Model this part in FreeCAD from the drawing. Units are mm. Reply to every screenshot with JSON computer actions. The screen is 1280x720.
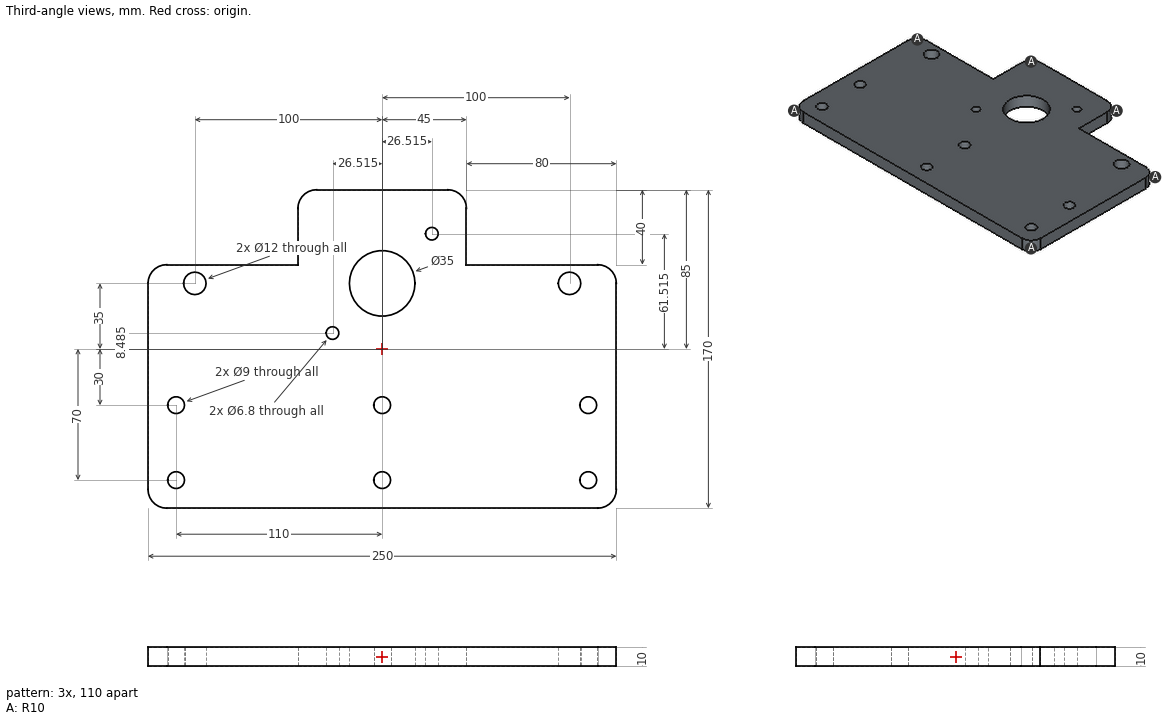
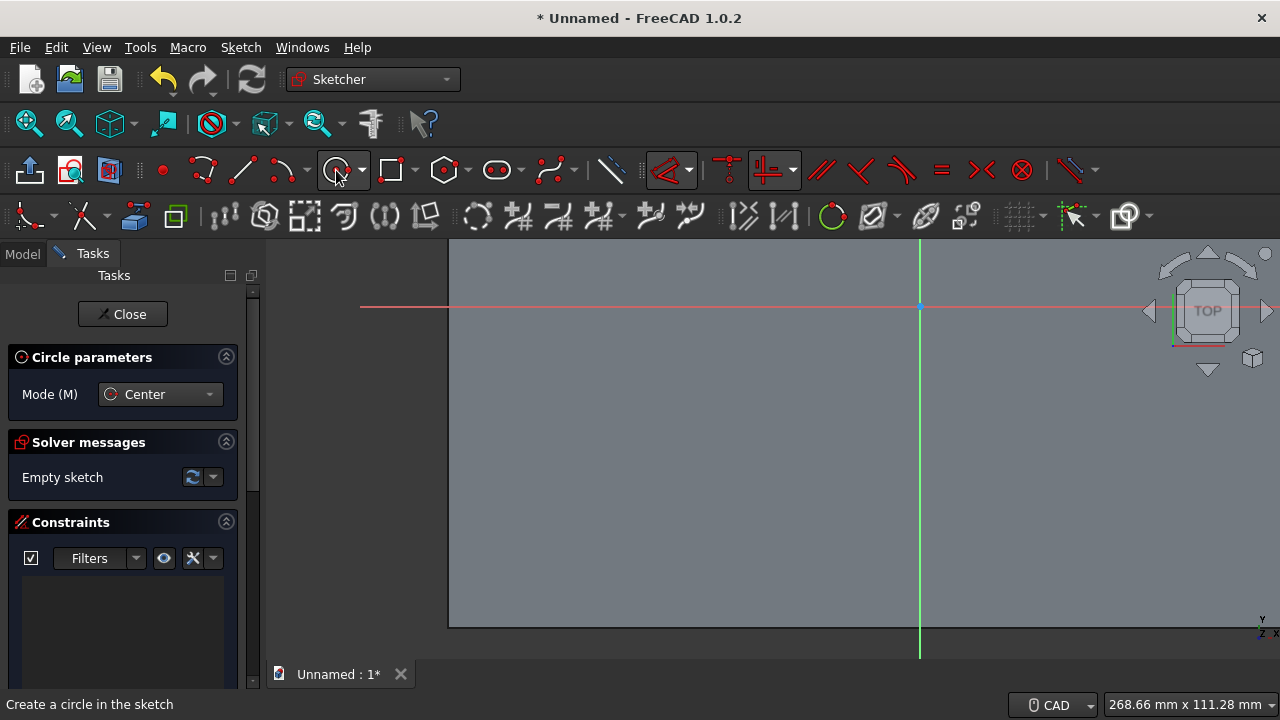
{"action": "scroll", "coordinate": [505, 420], "scroll_direction": "up", "scroll_amount": 2}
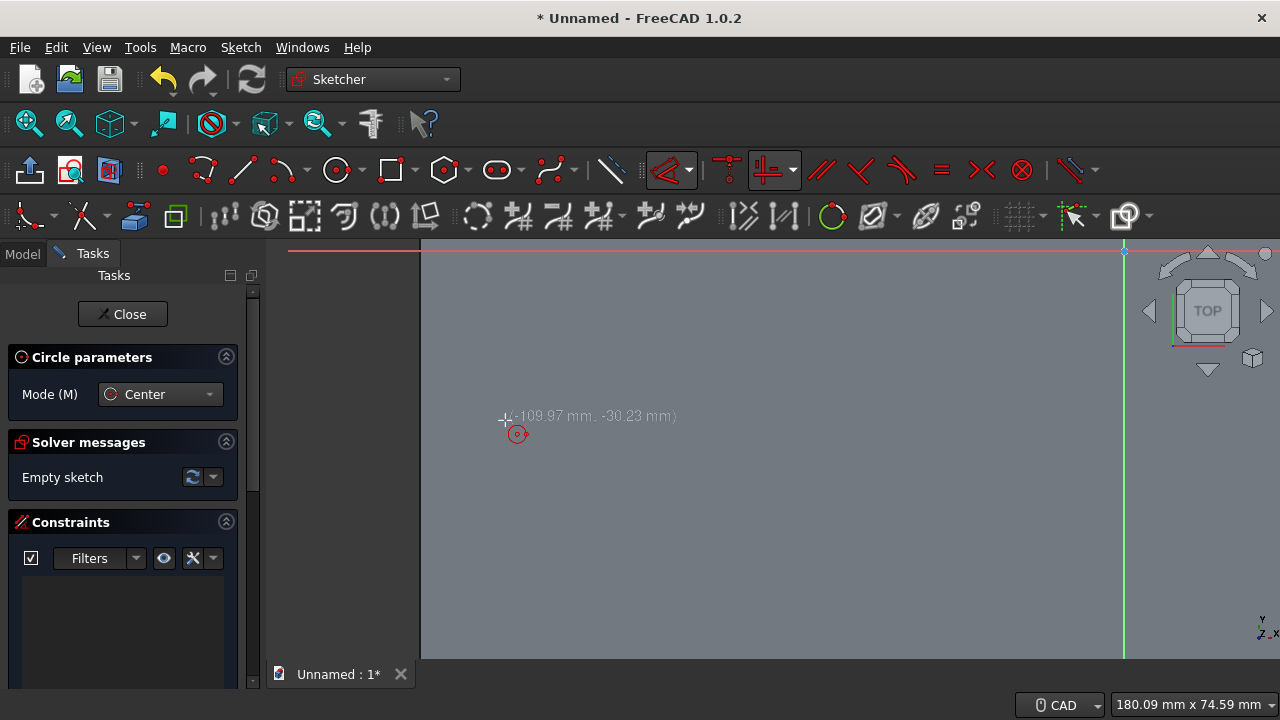
{"action": "left_click", "coordinate": [505, 420]}
{"action": "mouse_move", "coordinate": [523, 402]}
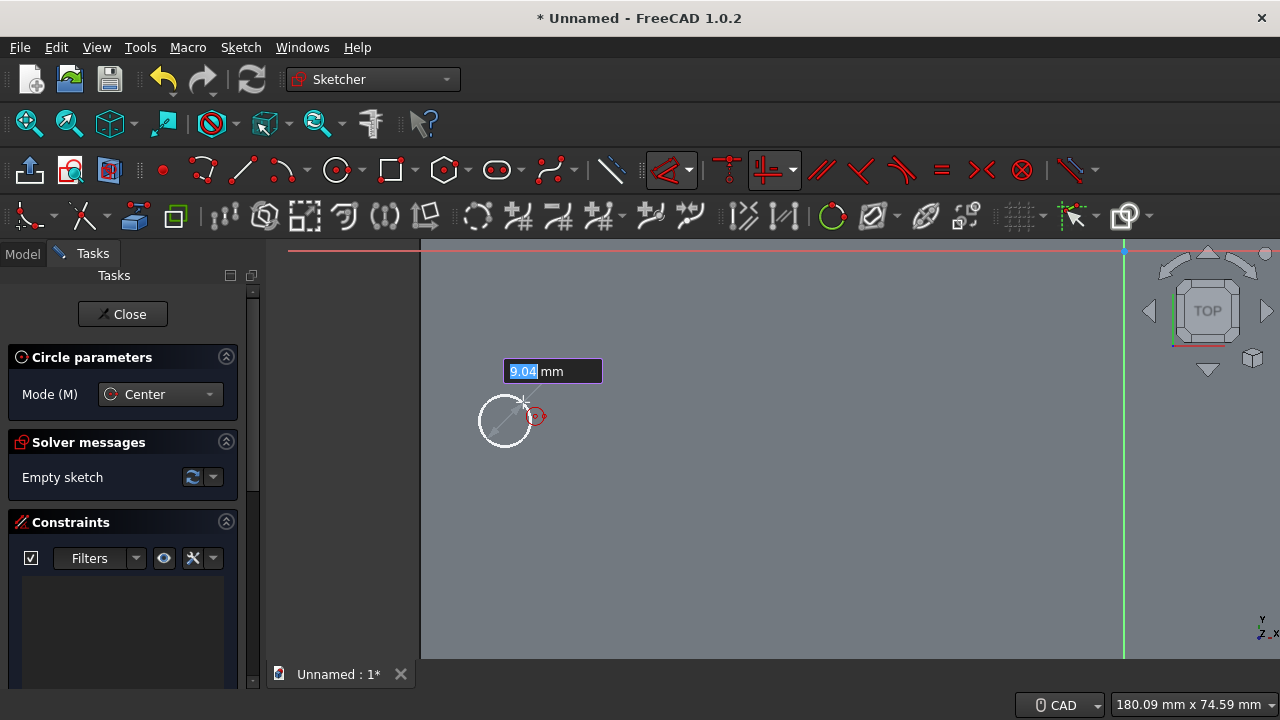
{"action": "type", "text": "9"}
{"action": "key", "text": "Return"}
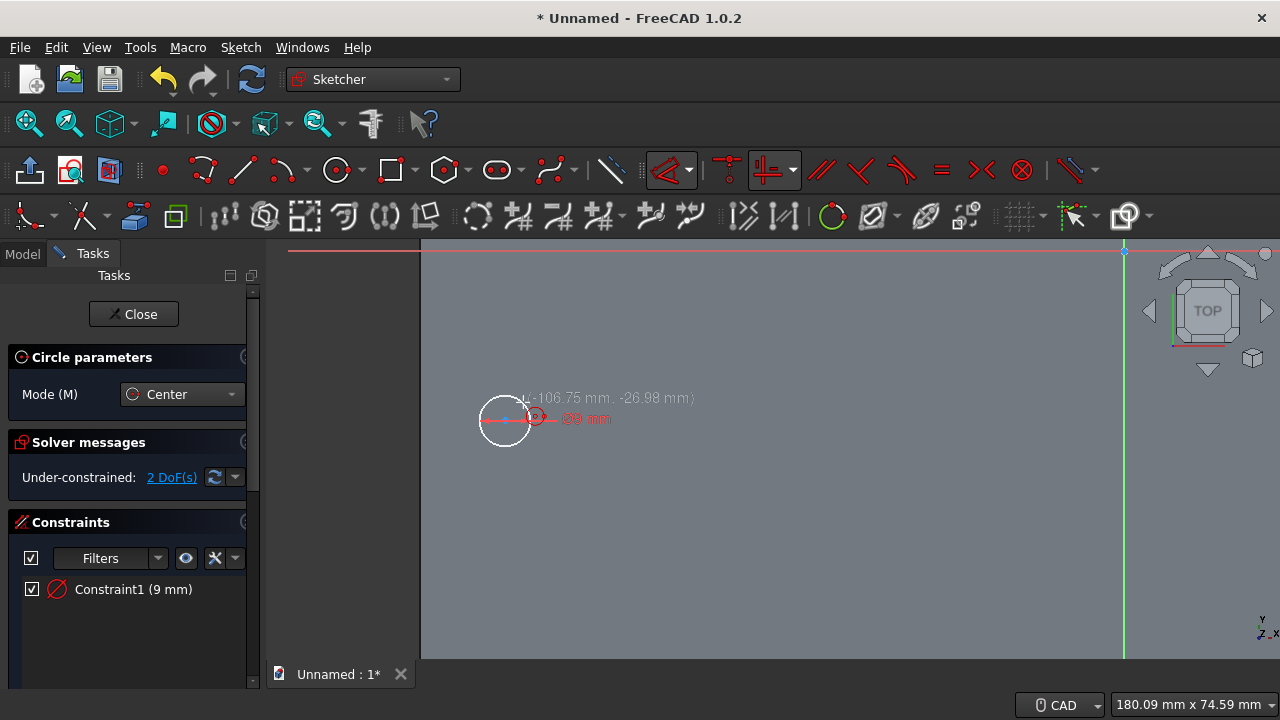
{"action": "scroll", "coordinate": [507, 425], "scroll_direction": "down", "scroll_amount": 2}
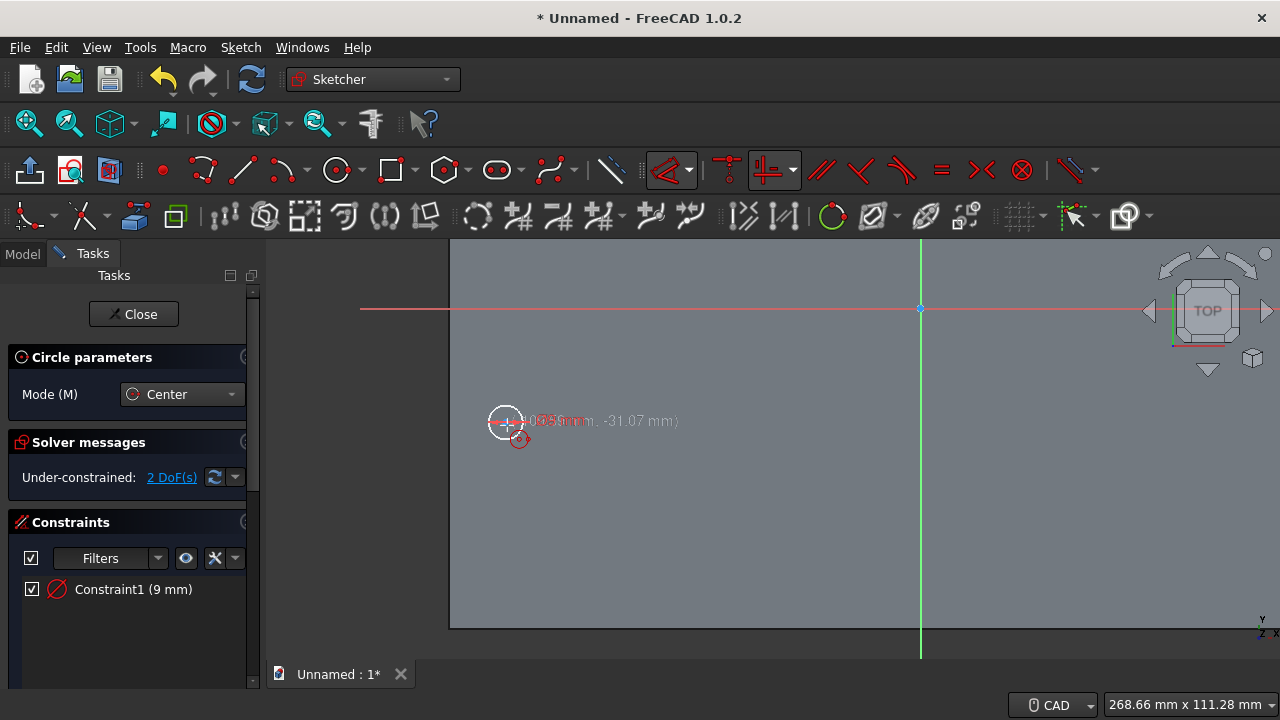
{"action": "scroll", "coordinate": [506, 573], "scroll_direction": "up", "scroll_amount": 2}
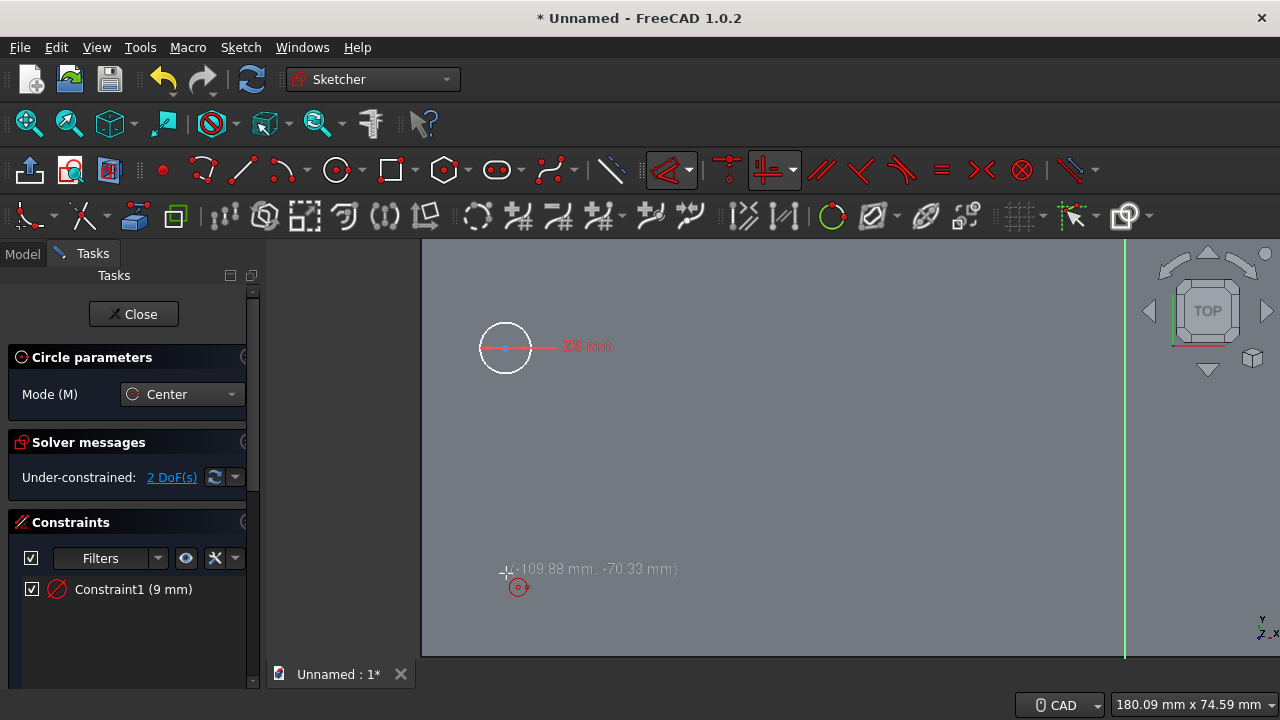
{"action": "left_click", "coordinate": [505, 572]}
{"action": "mouse_move", "coordinate": [523, 554]}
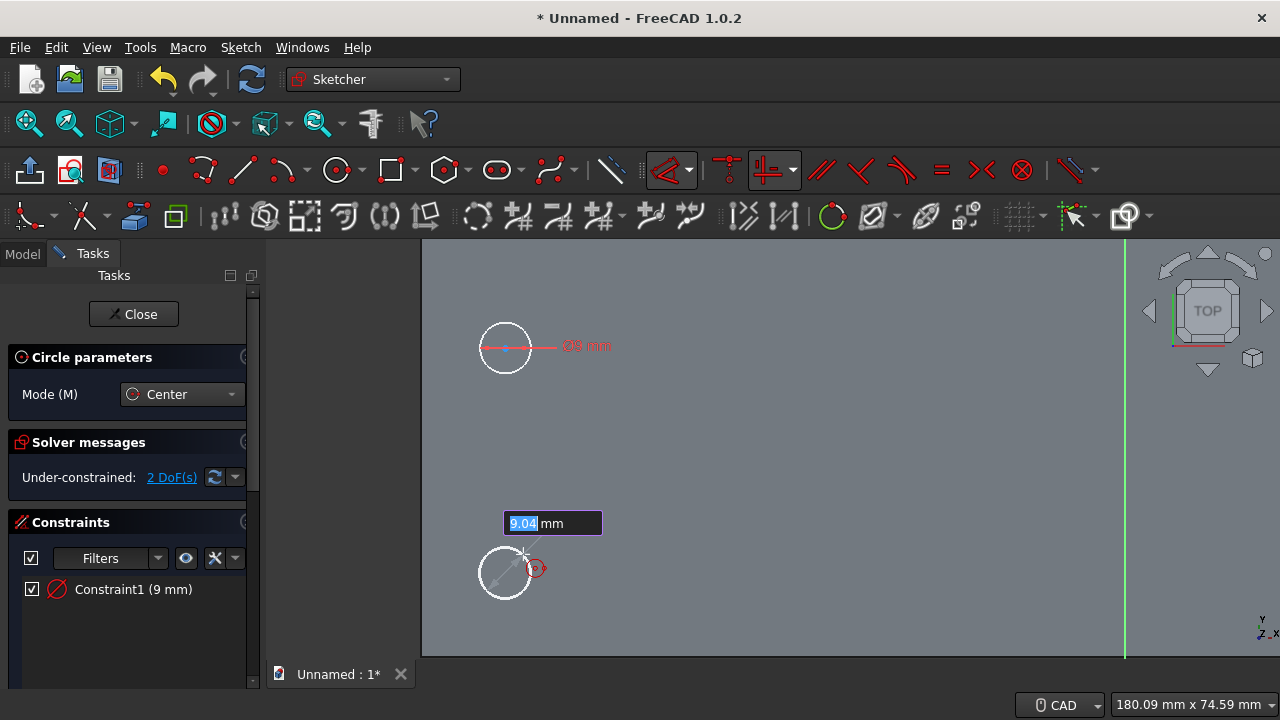
{"action": "type", "text": "9"}
{"action": "key", "text": "Return"}
{"action": "key", "text": "Escape"}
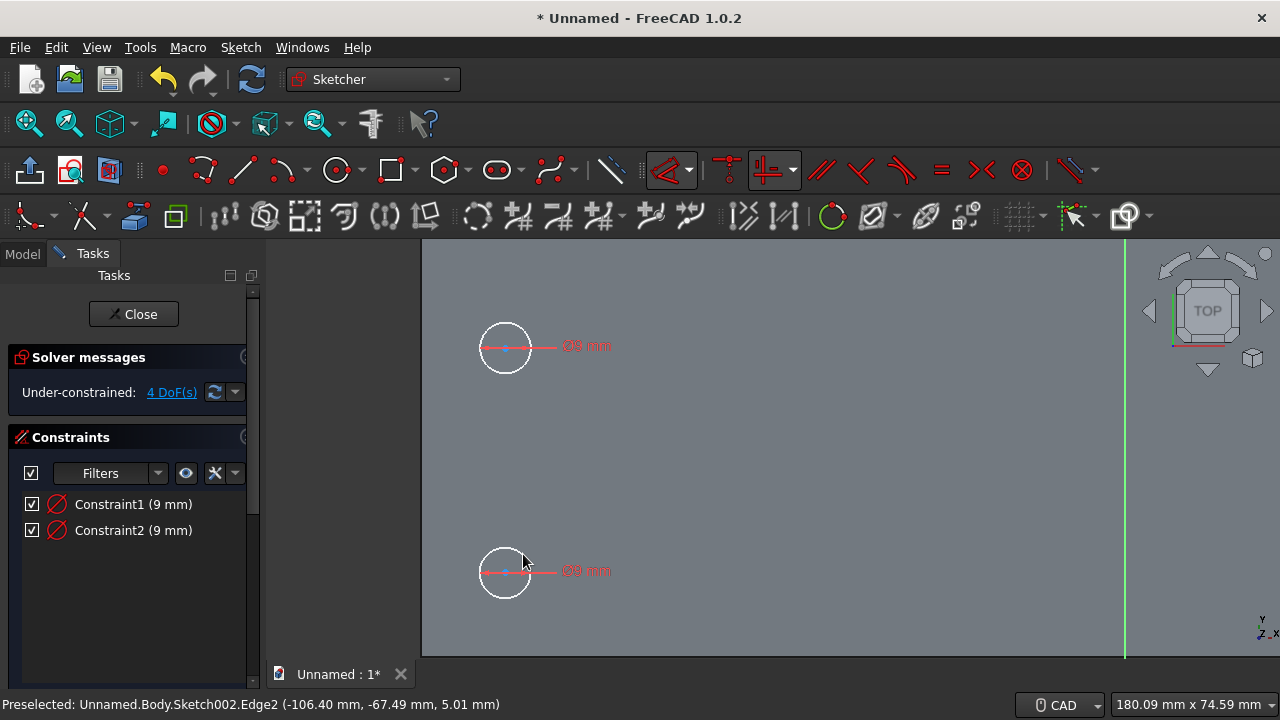
{"action": "left_click", "coordinate": [505, 348]}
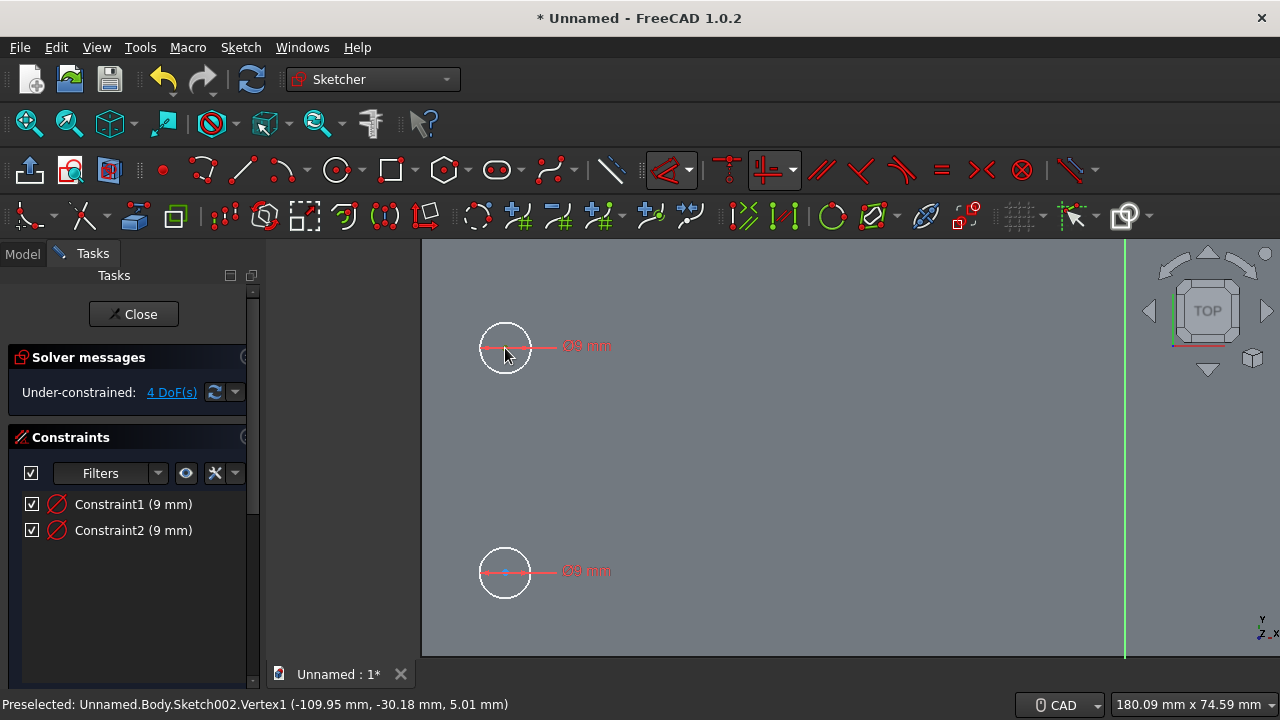
{"action": "left_click", "coordinate": [505, 573]}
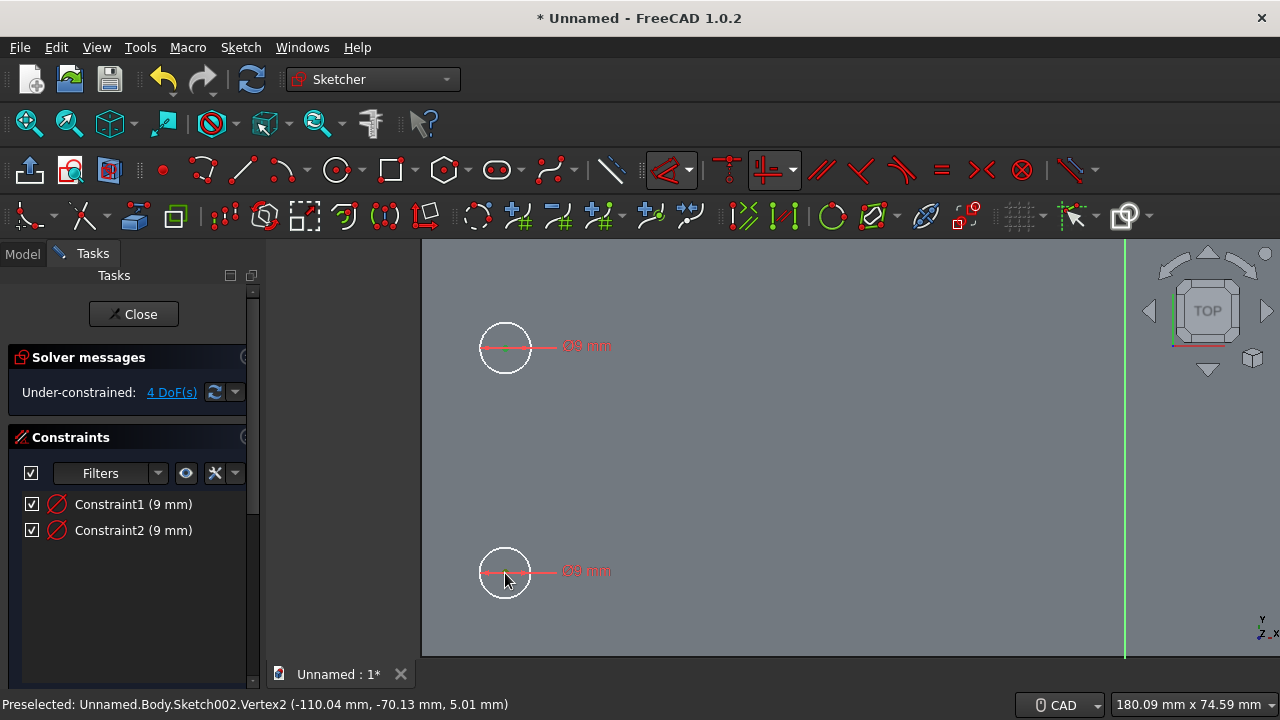
{"action": "key", "text": "v"}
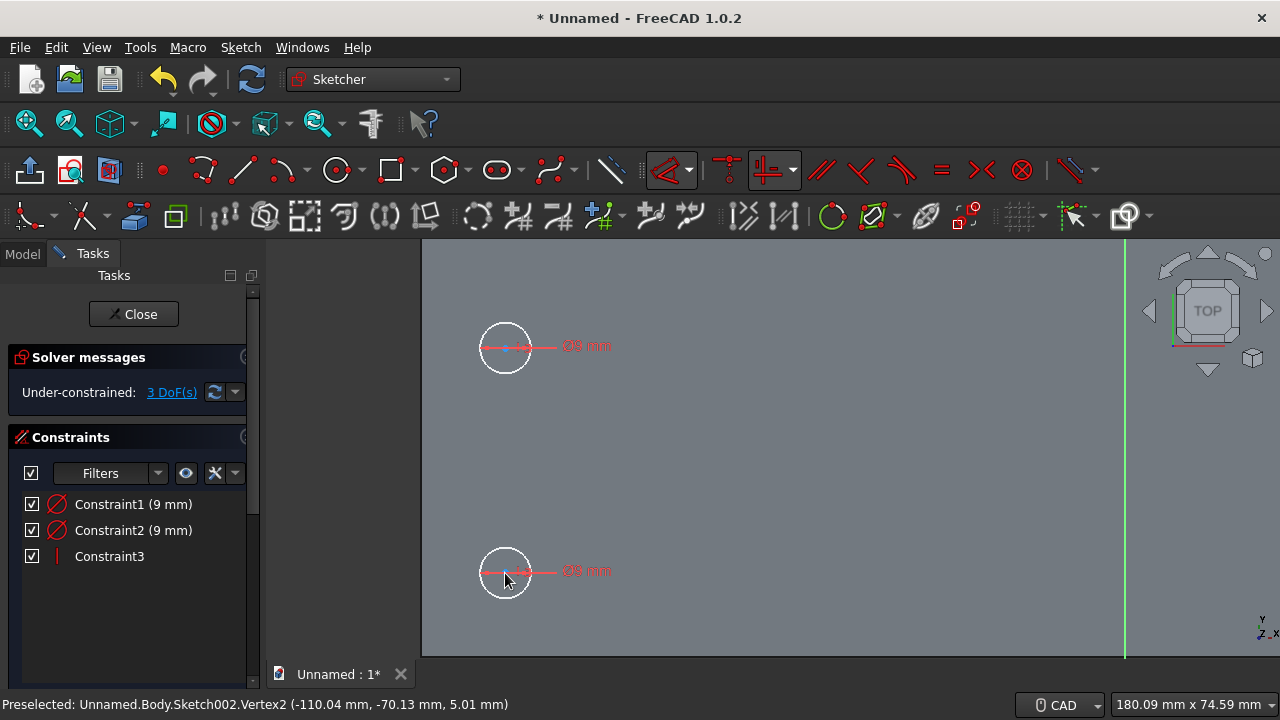
{"action": "left_click", "coordinate": [505, 348]}